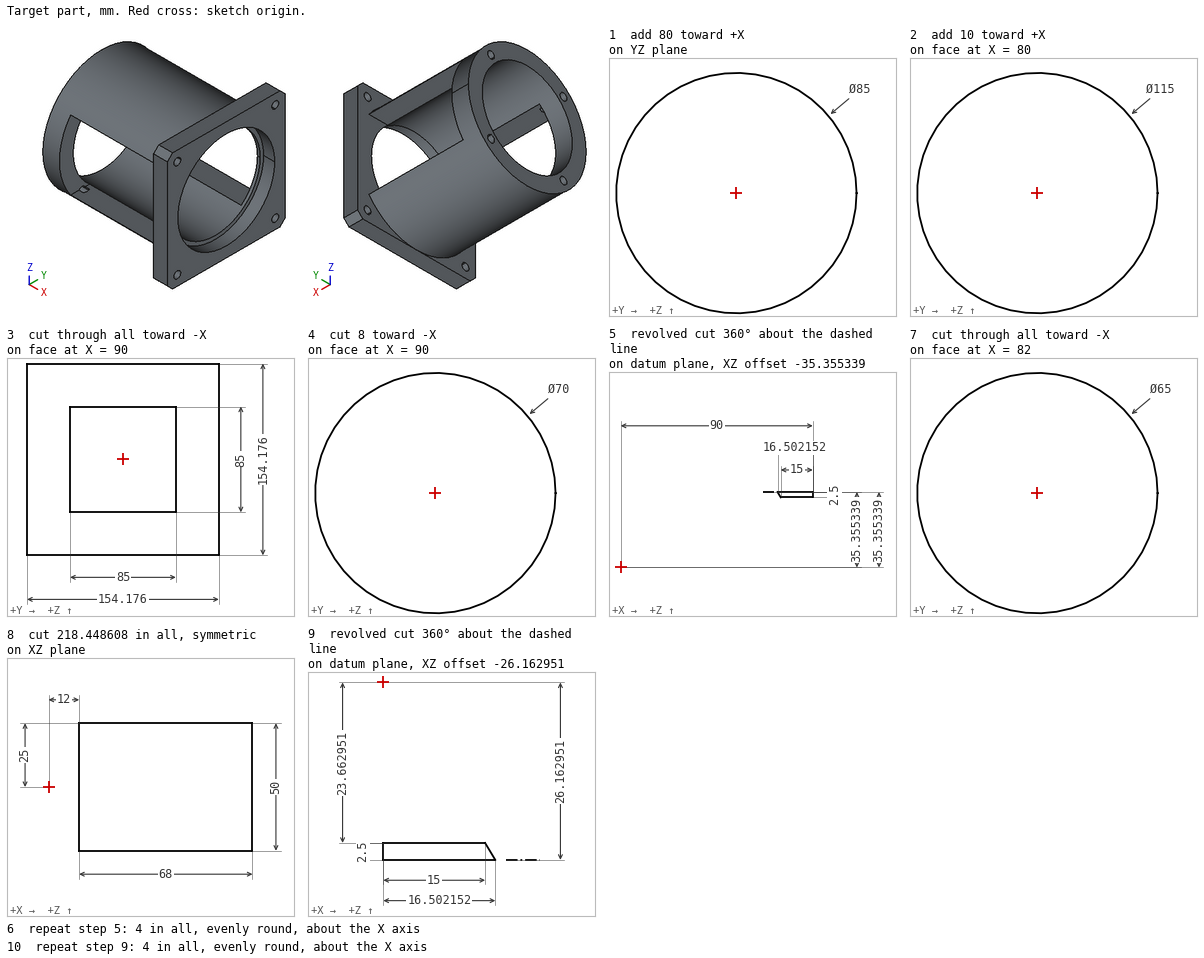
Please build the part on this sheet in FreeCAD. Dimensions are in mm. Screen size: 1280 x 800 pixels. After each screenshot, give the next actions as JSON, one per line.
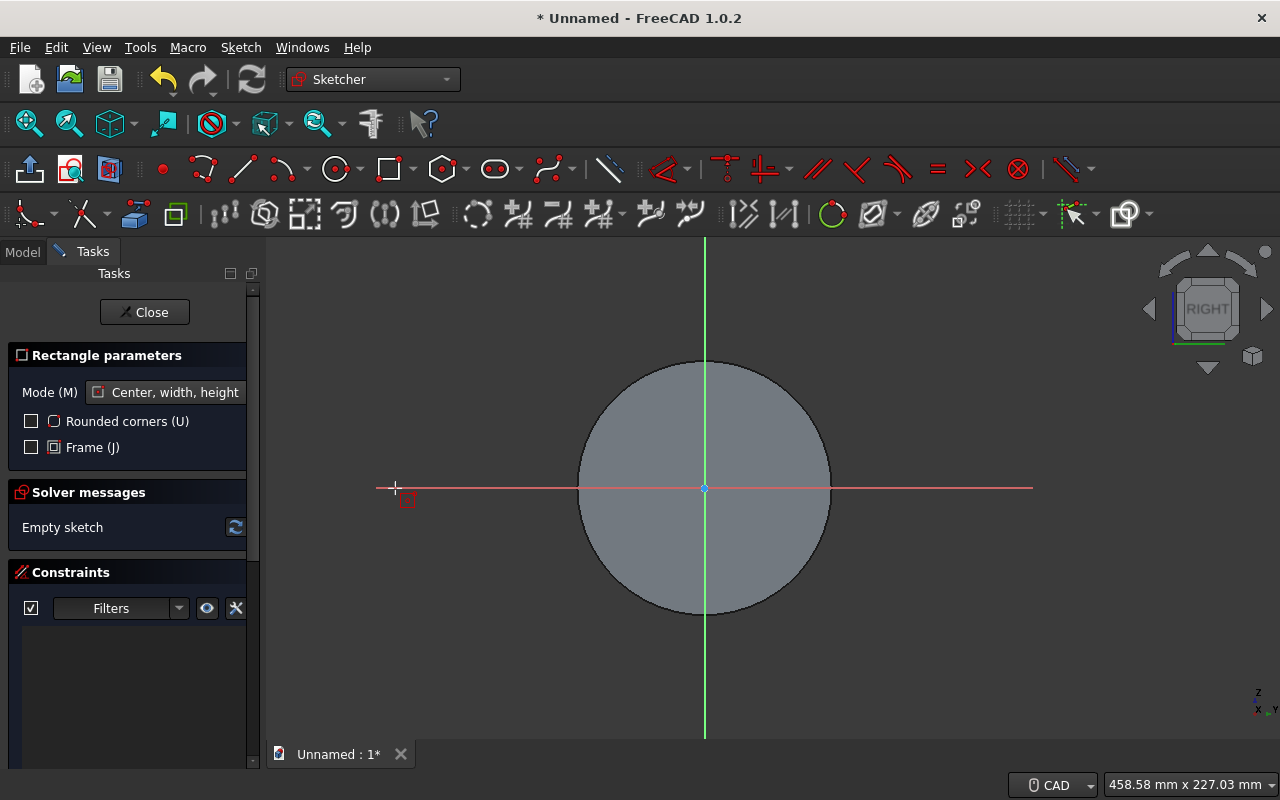
{"action": "left_click", "coordinate": [705, 488]}
{"action": "mouse_move", "coordinate": [875, 318]}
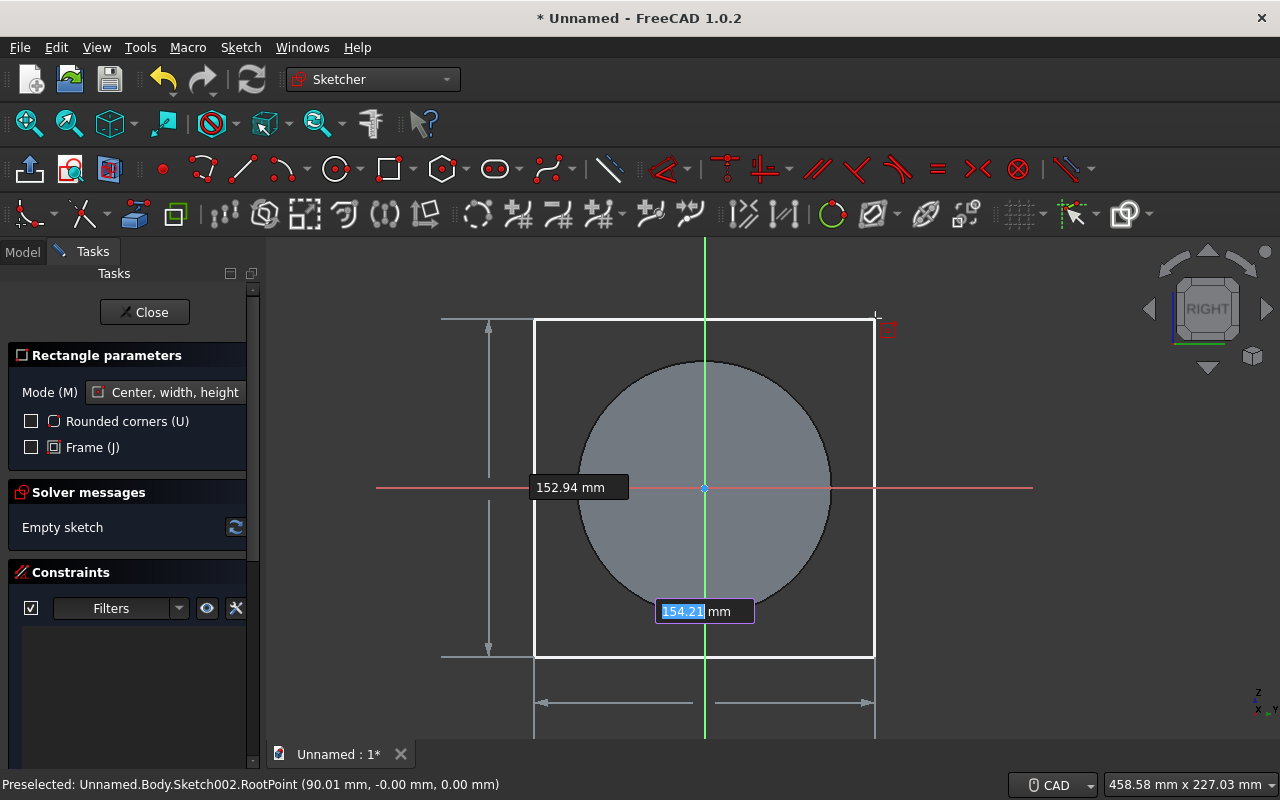
{"action": "type", "text": "154.176"}
{"action": "key", "text": "Tab"}
{"action": "type", "text": "154.176"}
{"action": "key", "text": "Return"}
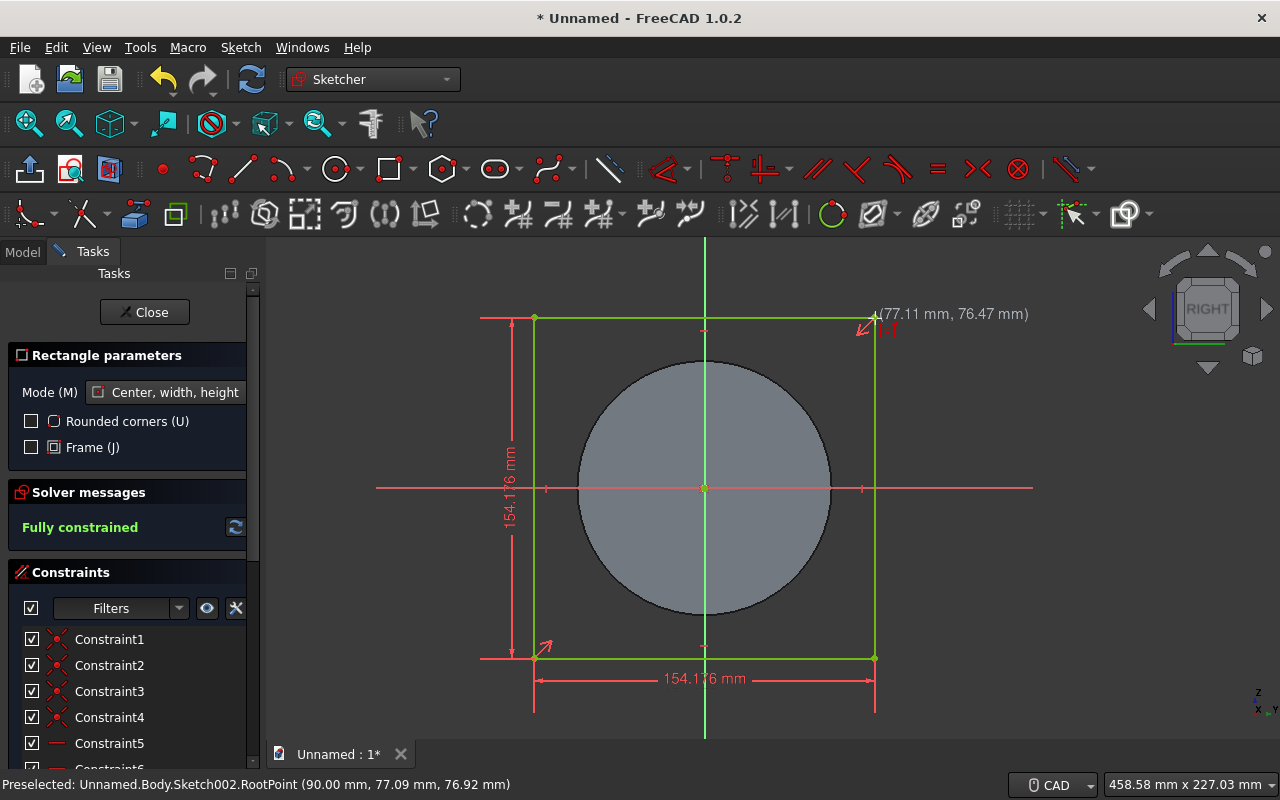
{"action": "left_click", "coordinate": [705, 488]}
{"action": "mouse_move", "coordinate": [798, 394]}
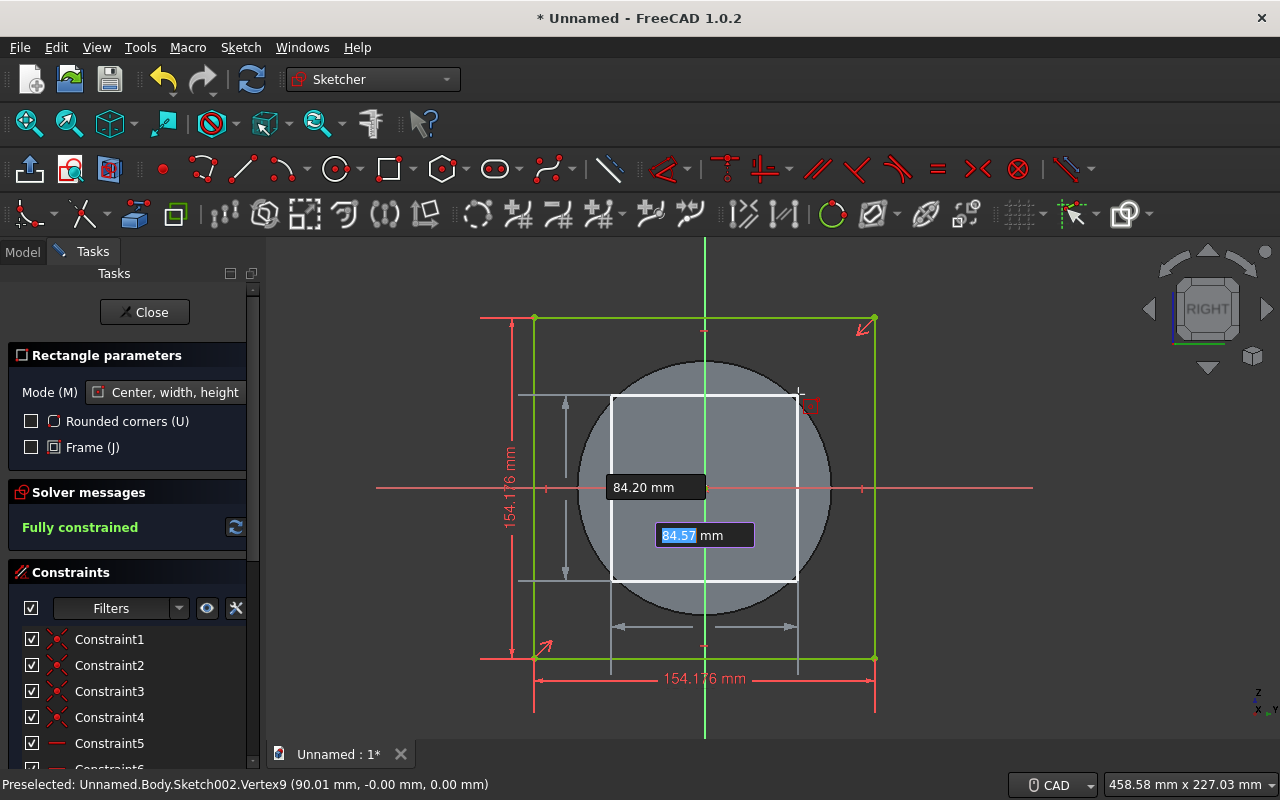
{"action": "type", "text": "85"}
{"action": "key", "text": "Tab"}
{"action": "type", "text": "85"}
{"action": "key", "text": "Return"}
{"action": "key", "text": "Escape"}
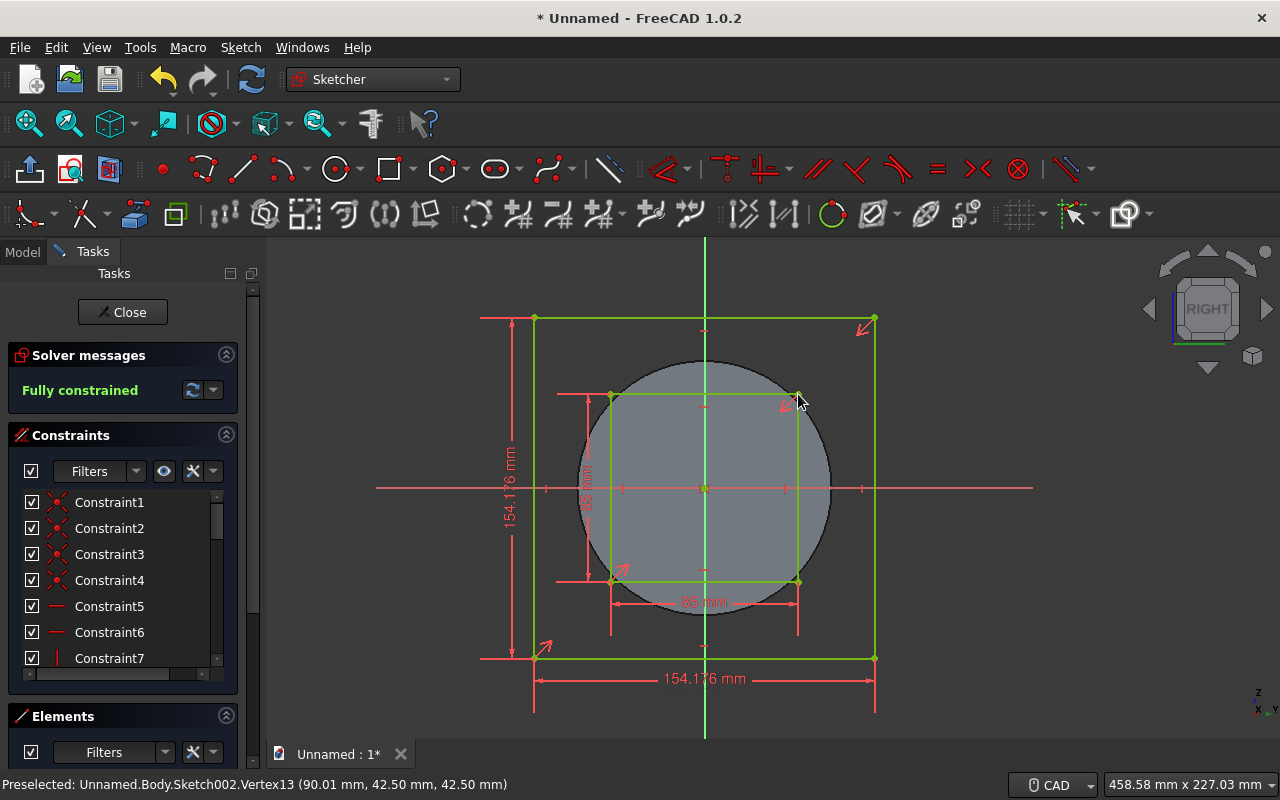
{"action": "left_click", "coordinate": [123, 312]}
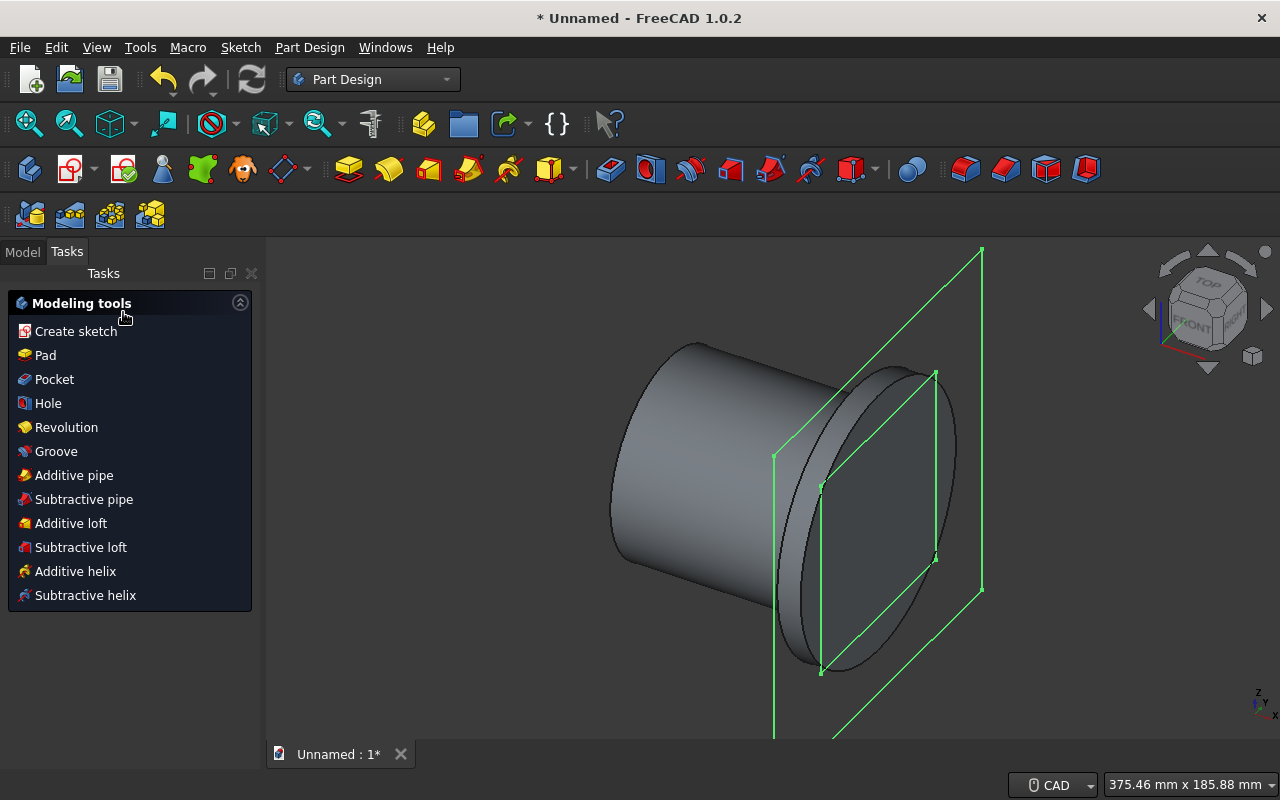
{"action": "left_click", "coordinate": [612, 170]}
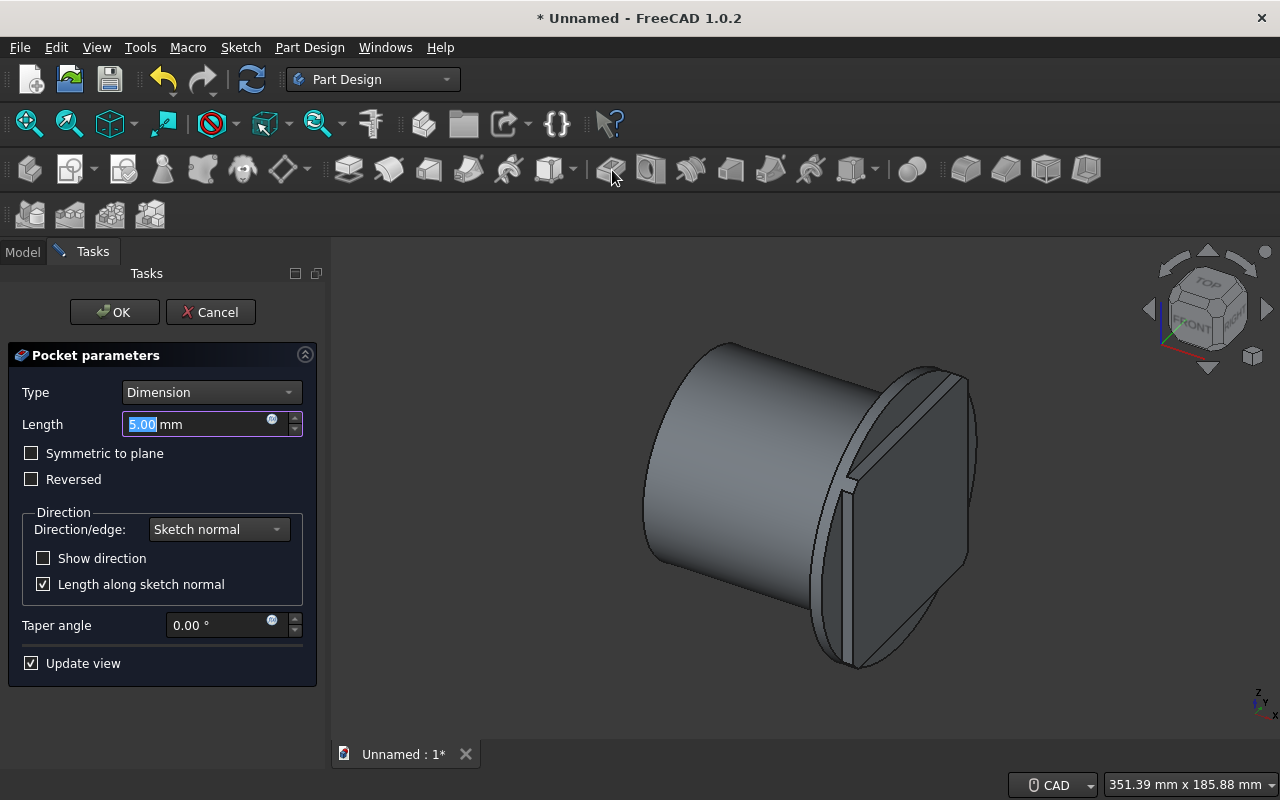
{"action": "left_click", "coordinate": [212, 392]}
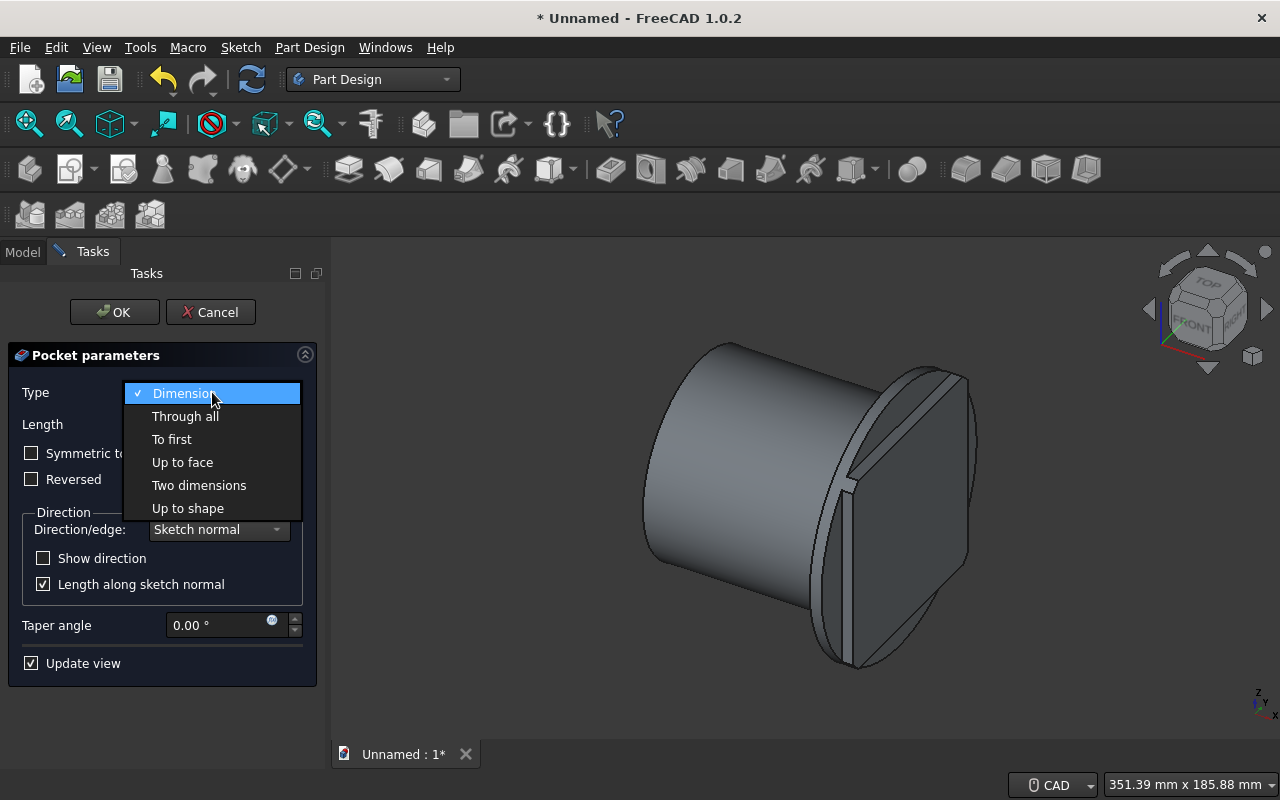
{"action": "left_click", "coordinate": [212, 416]}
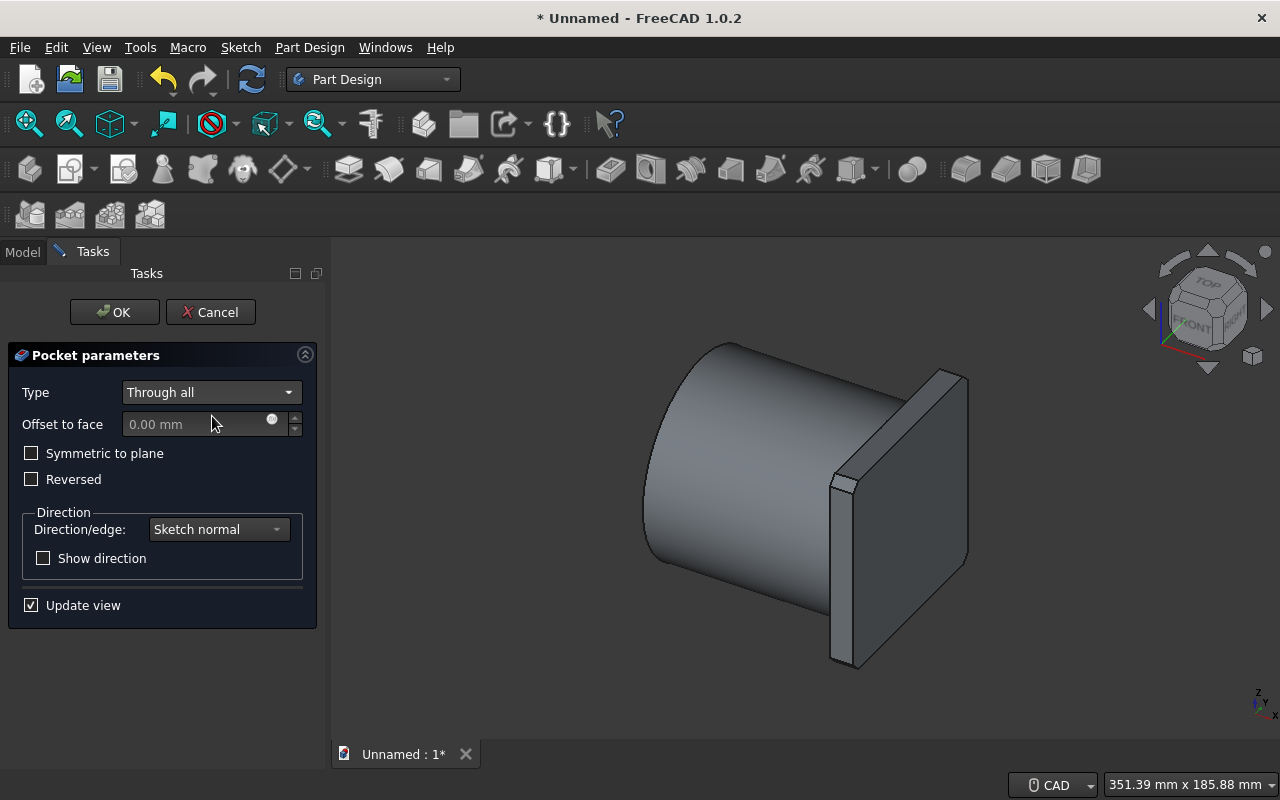
{"action": "left_click", "coordinate": [115, 312]}